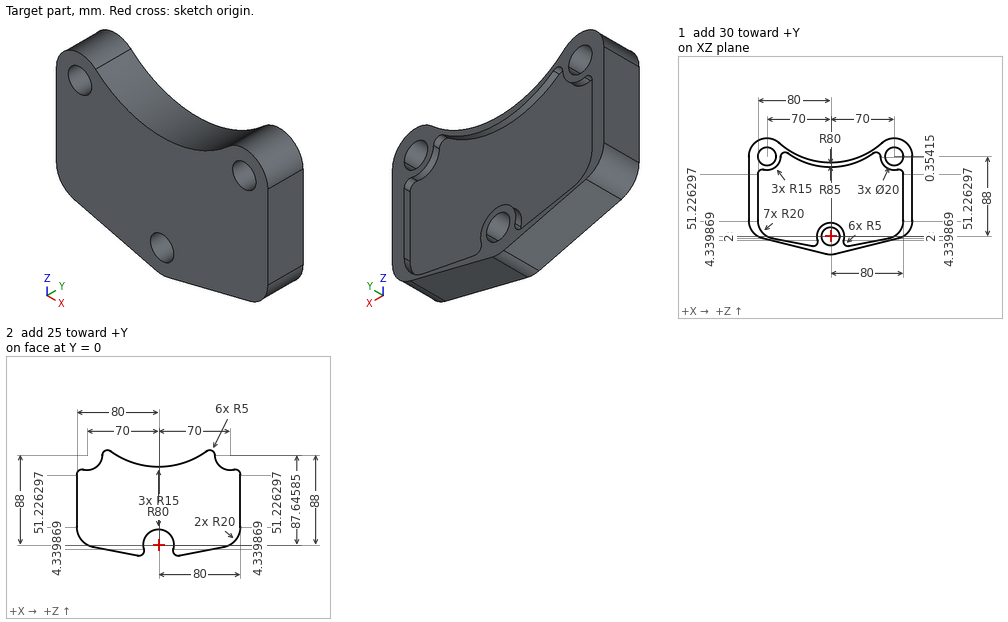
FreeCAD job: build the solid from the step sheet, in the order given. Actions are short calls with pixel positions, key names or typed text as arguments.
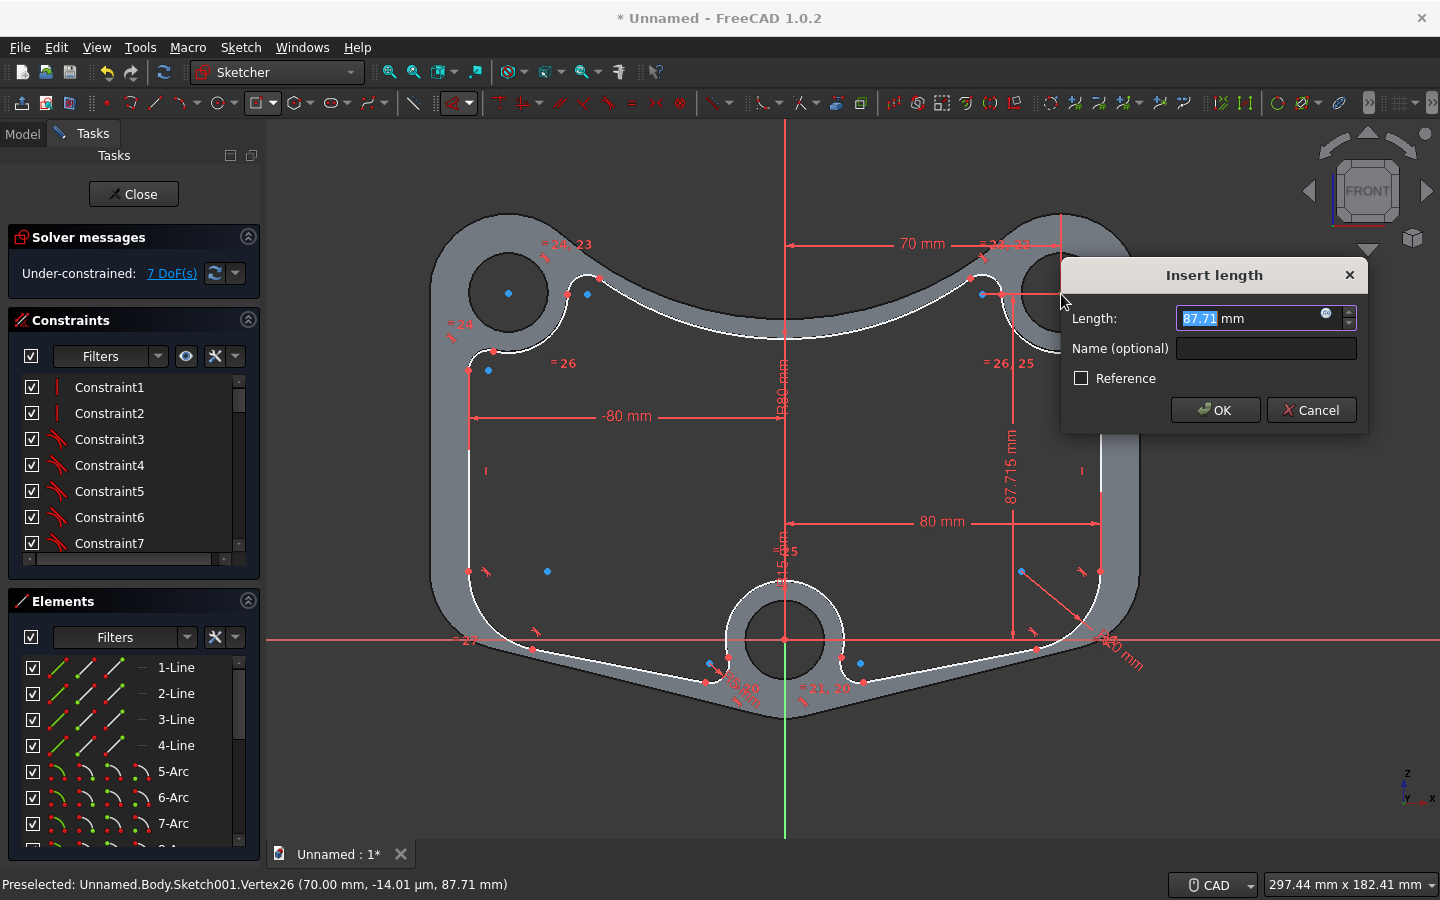
text(88)
key(Return)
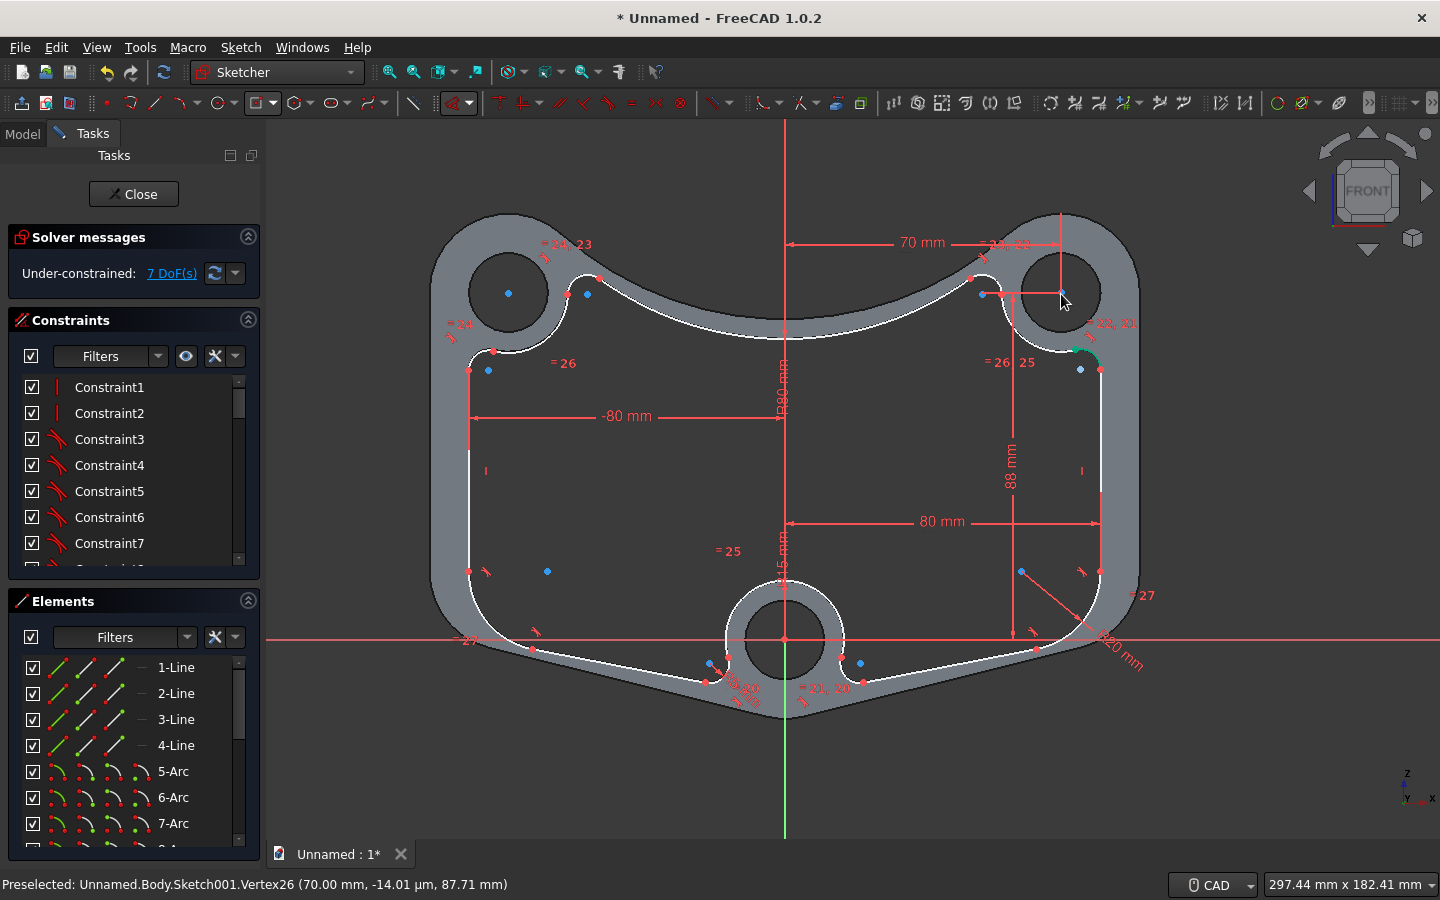
click(509, 294)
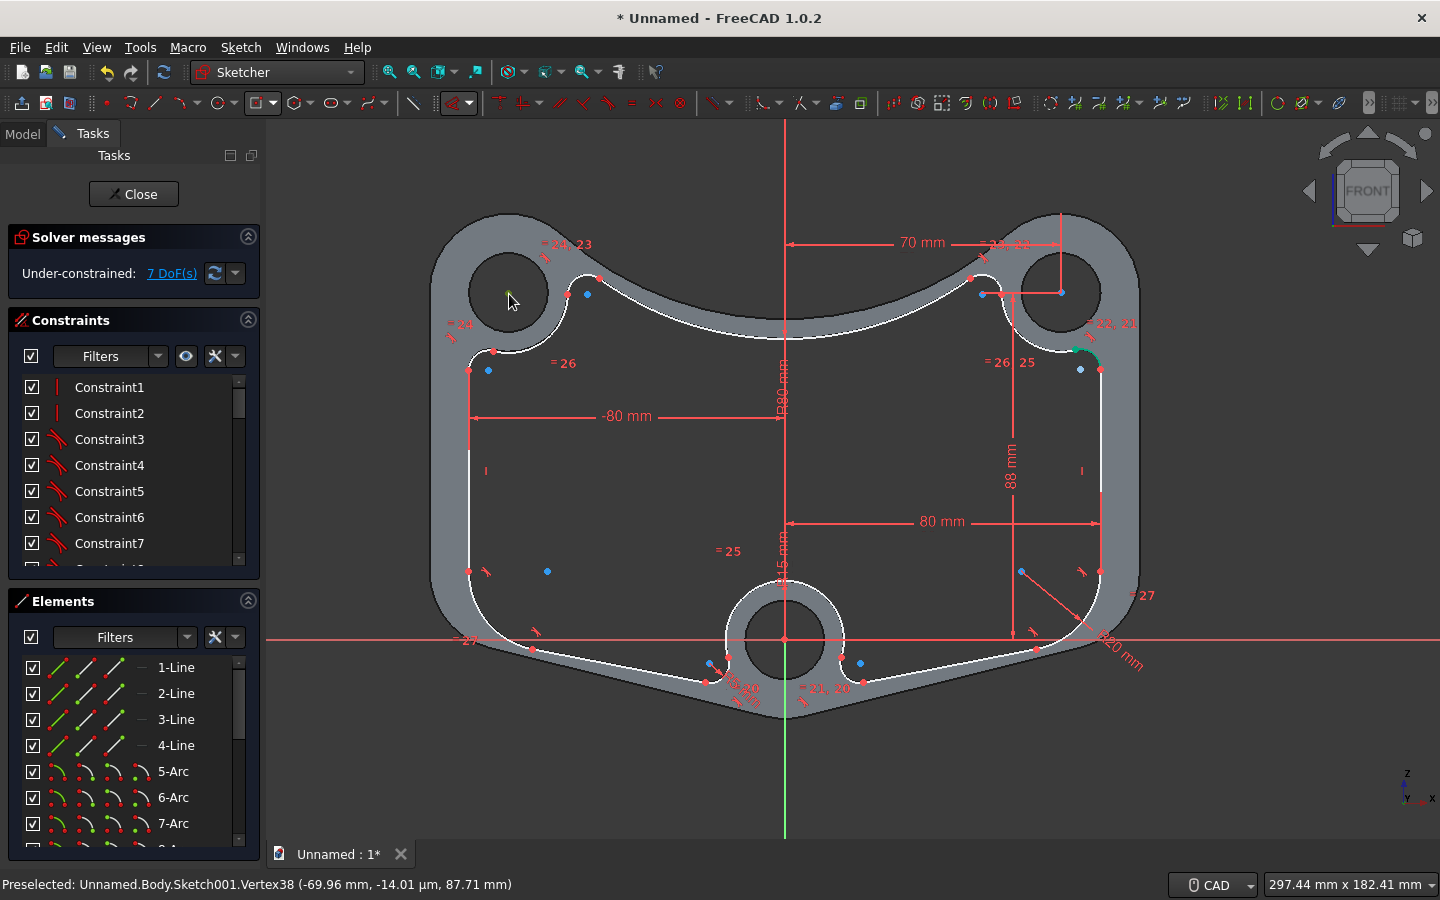
key(l)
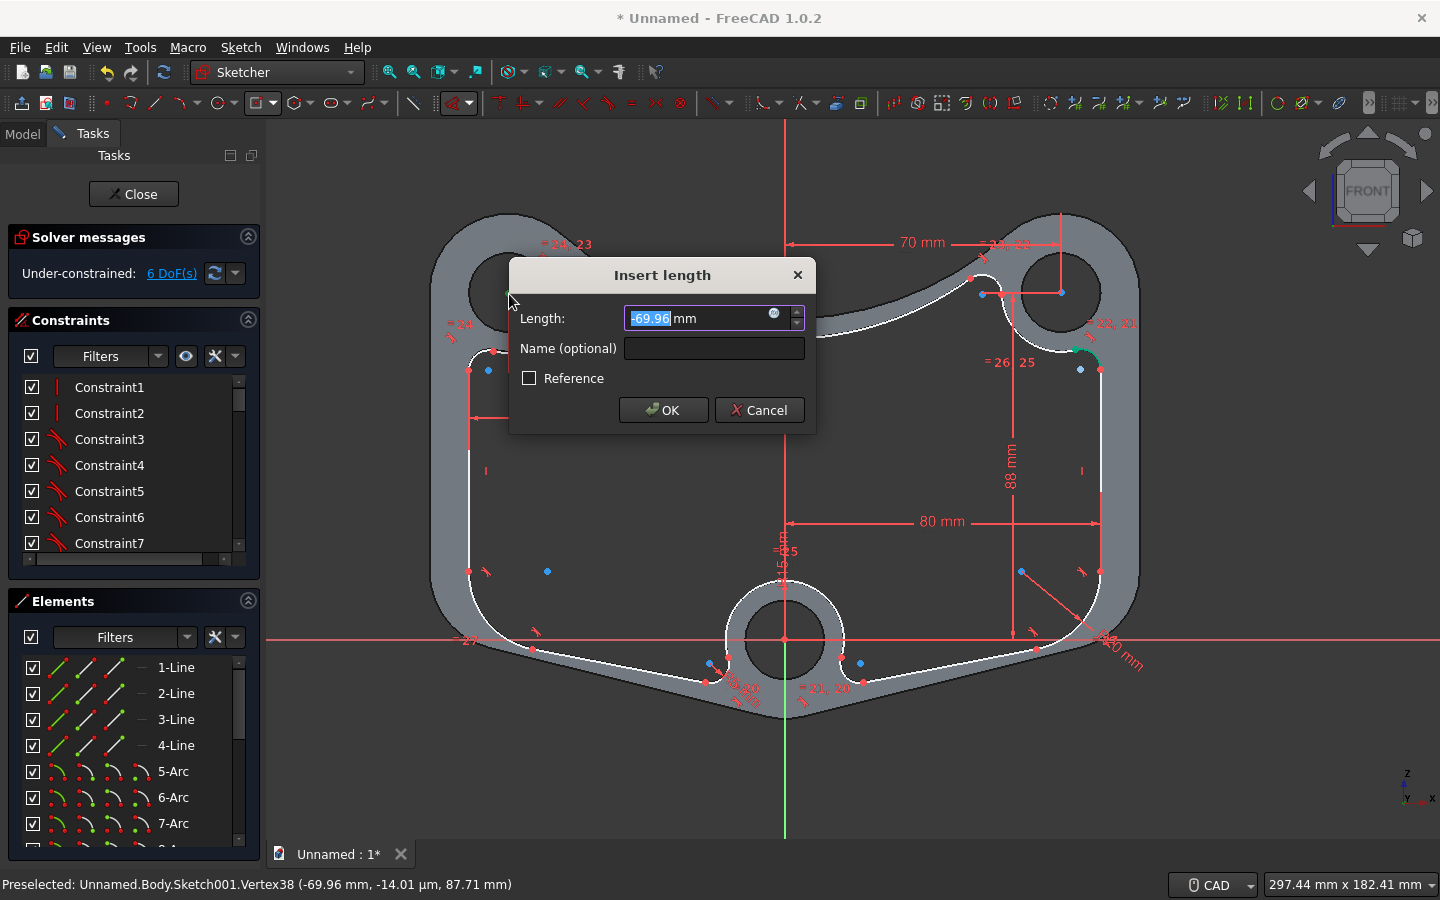
text(-70)
key(Return)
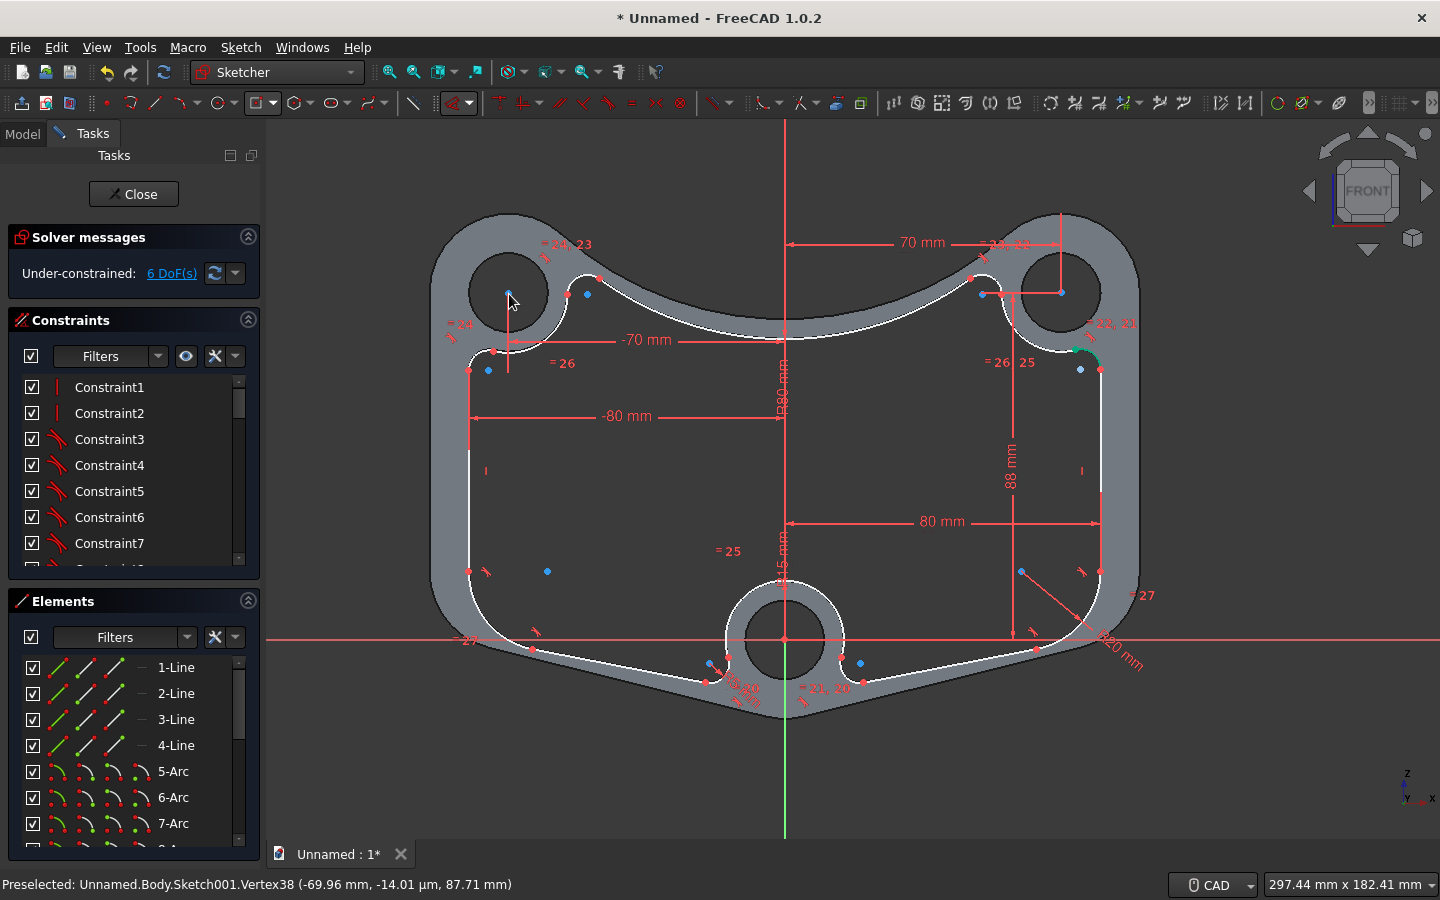
click(508, 294)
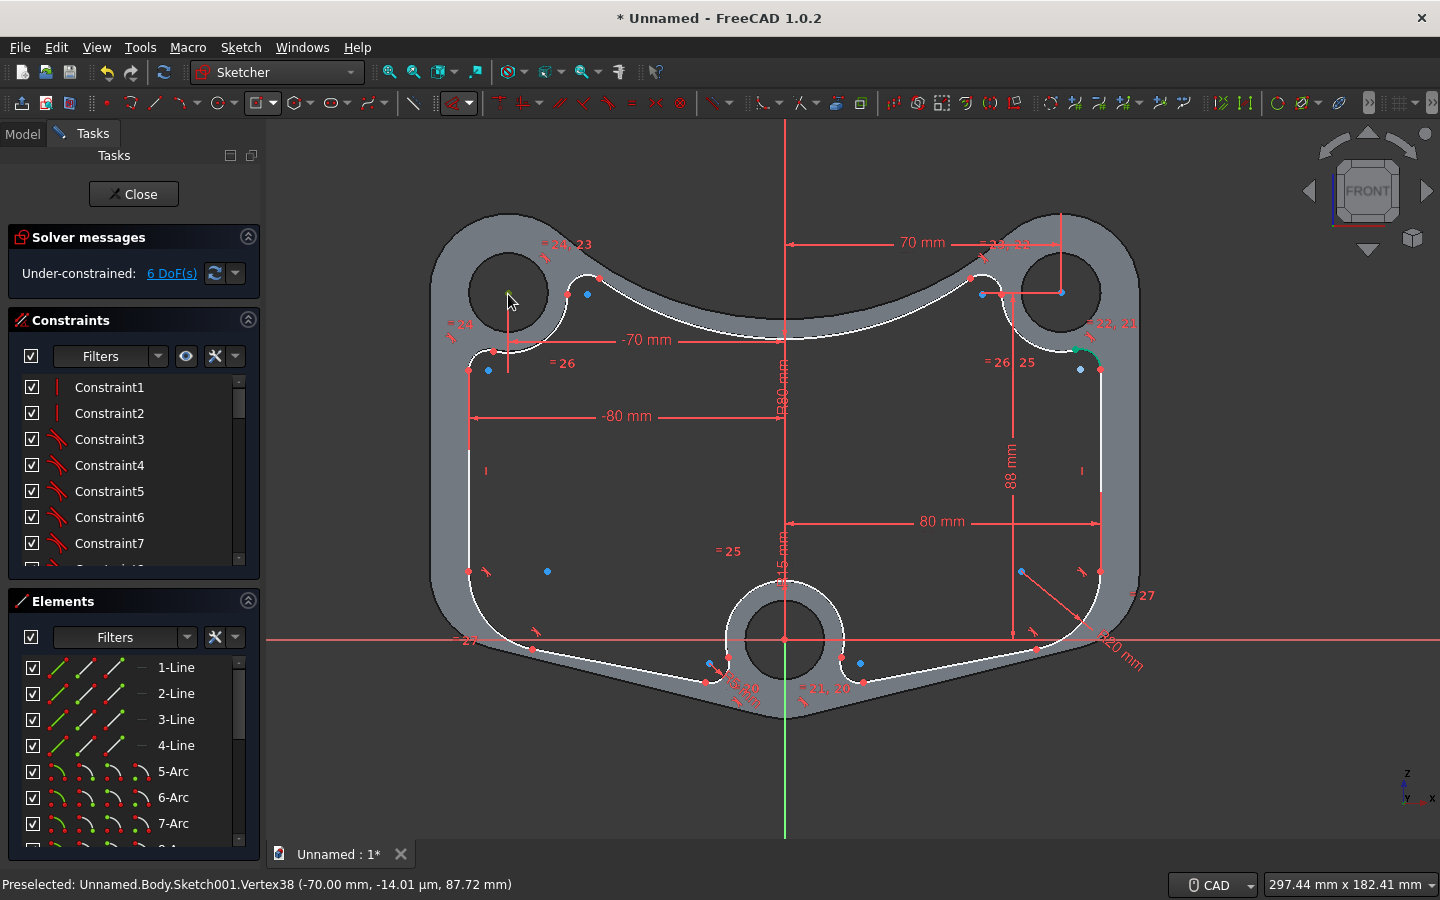
click(472, 104)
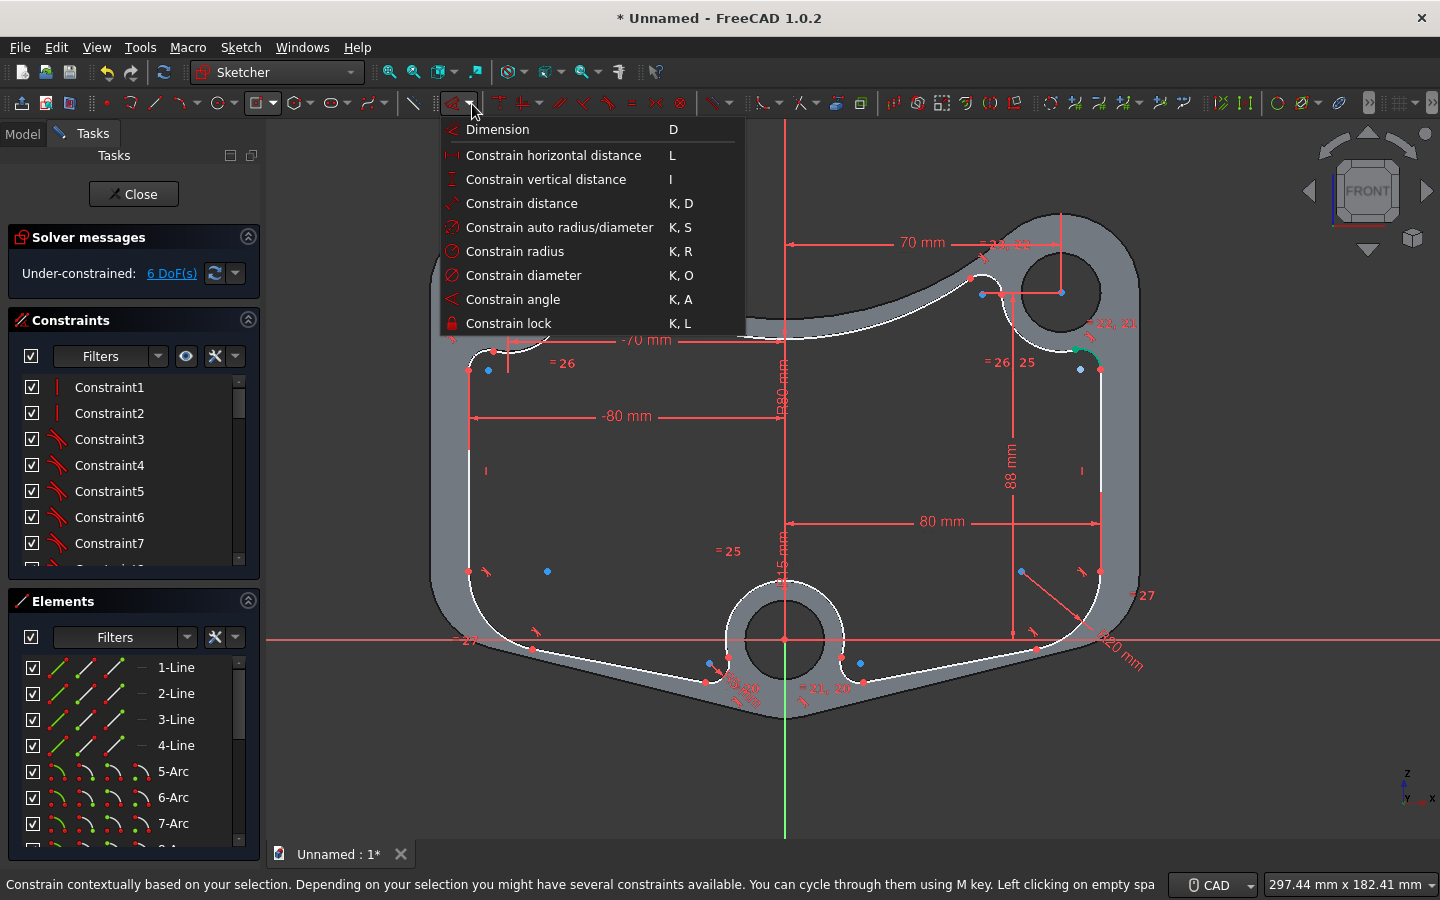
click(593, 179)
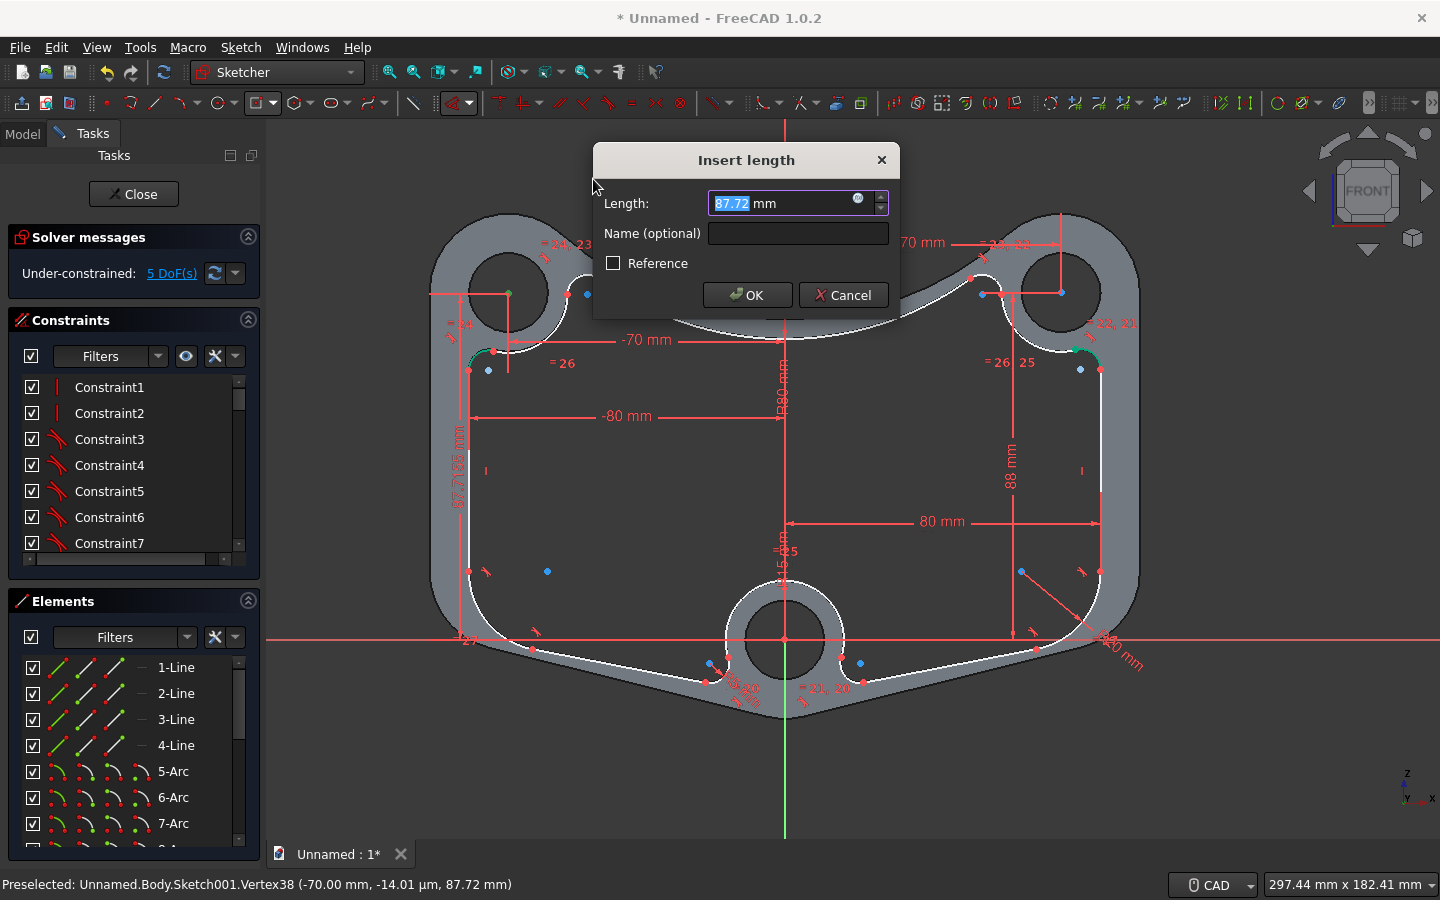
text(88)
key(Return)